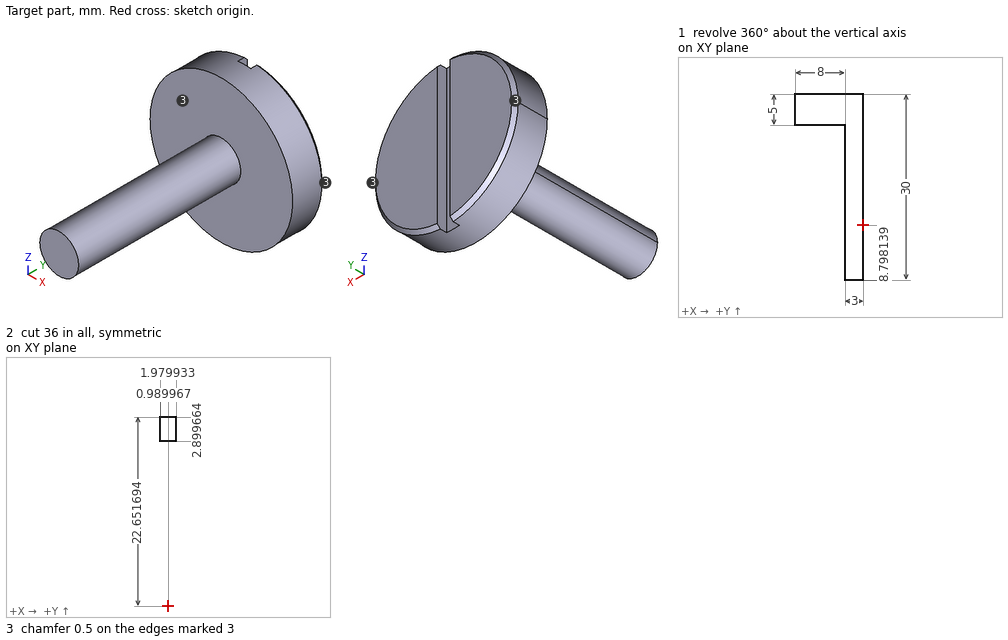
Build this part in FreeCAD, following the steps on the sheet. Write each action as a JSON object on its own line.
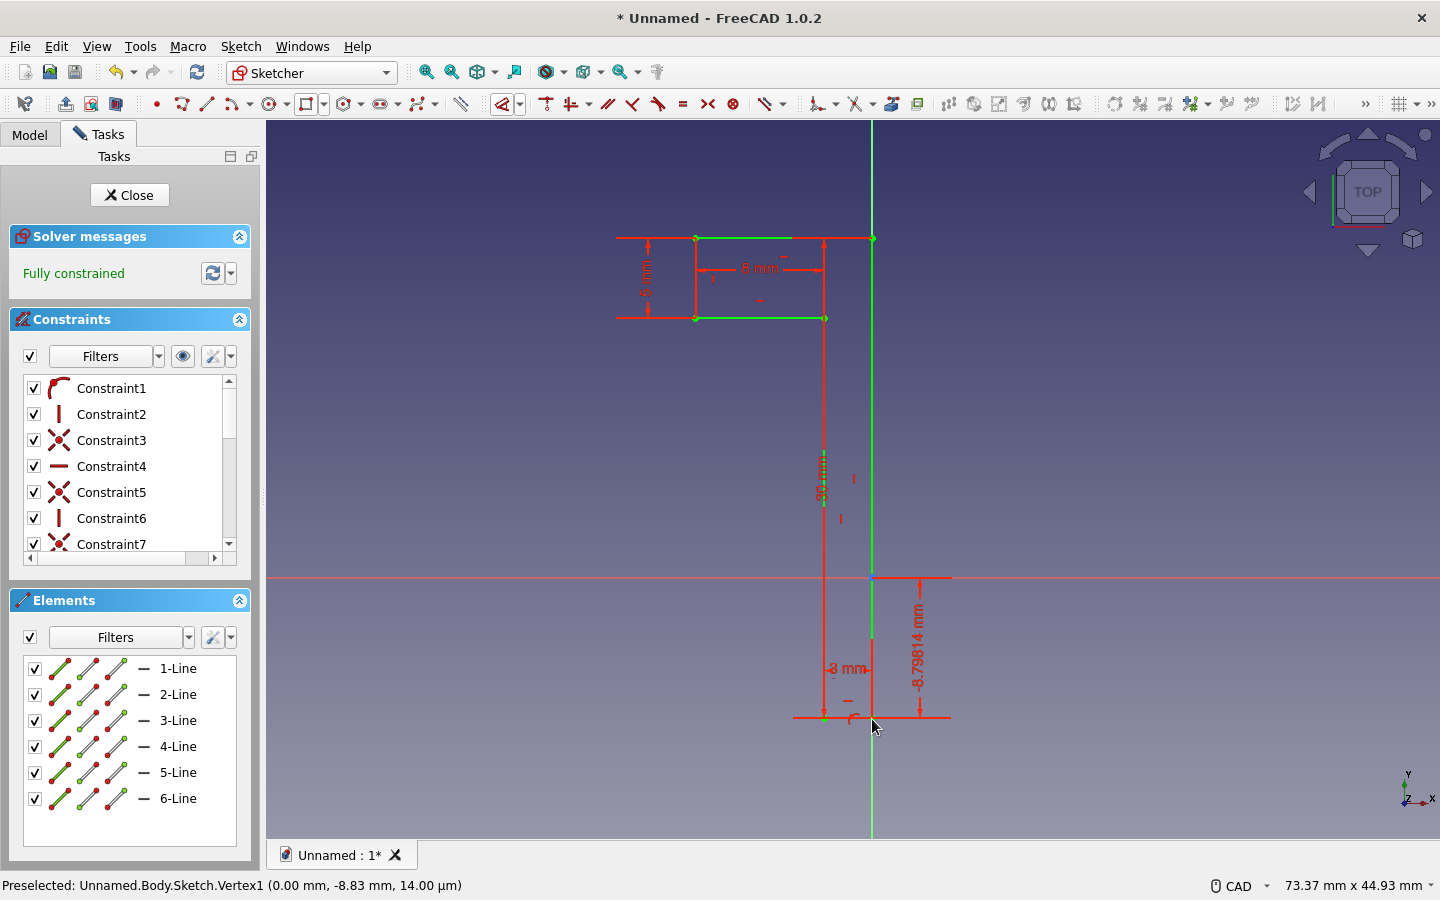
{"action": "left_click", "coordinate": [130, 195]}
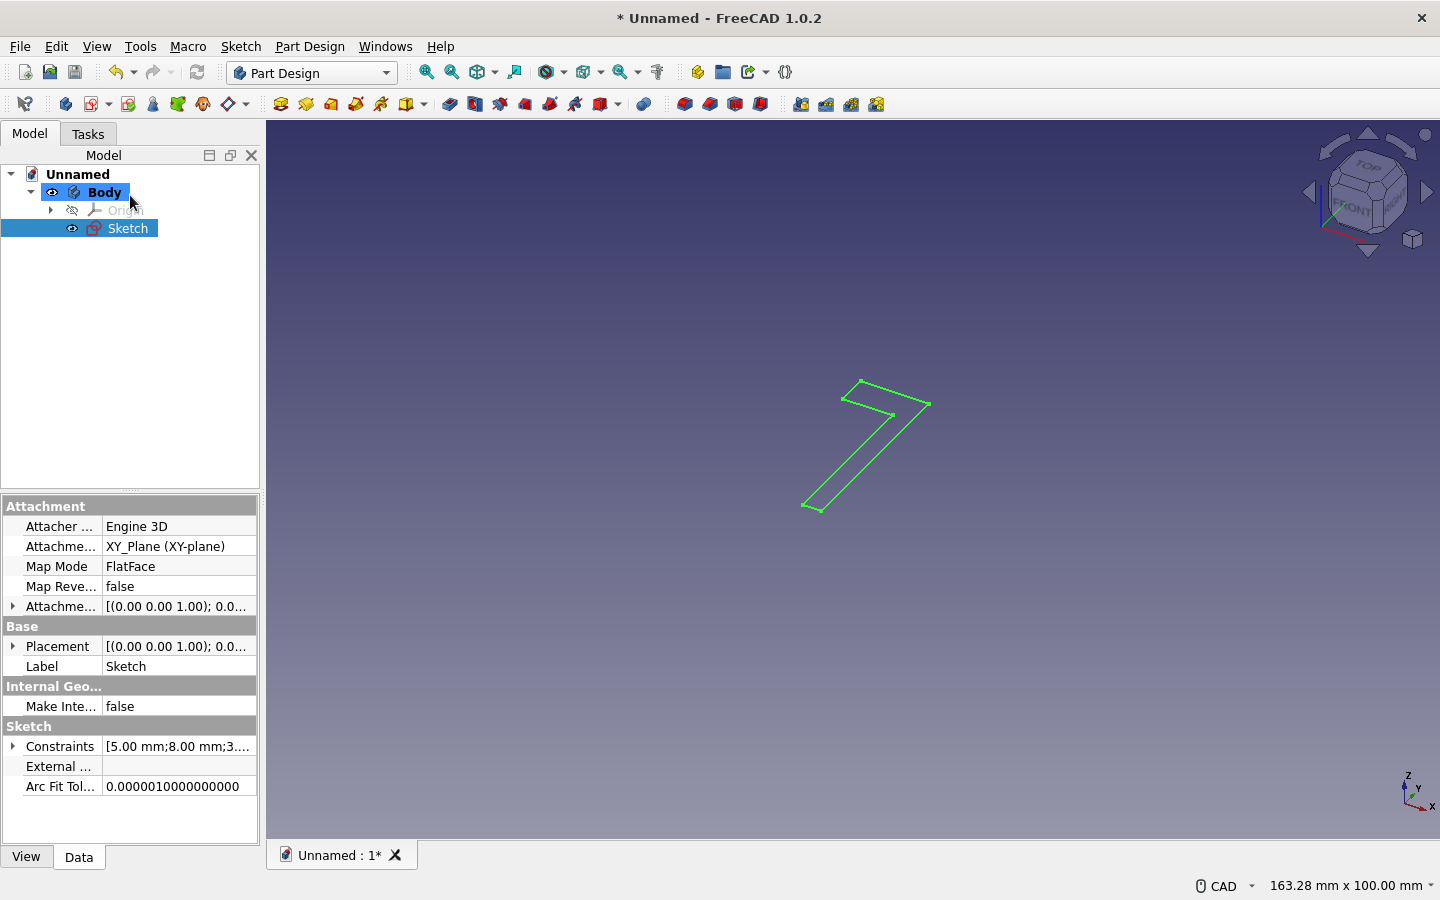
{"action": "left_click", "coordinate": [306, 104]}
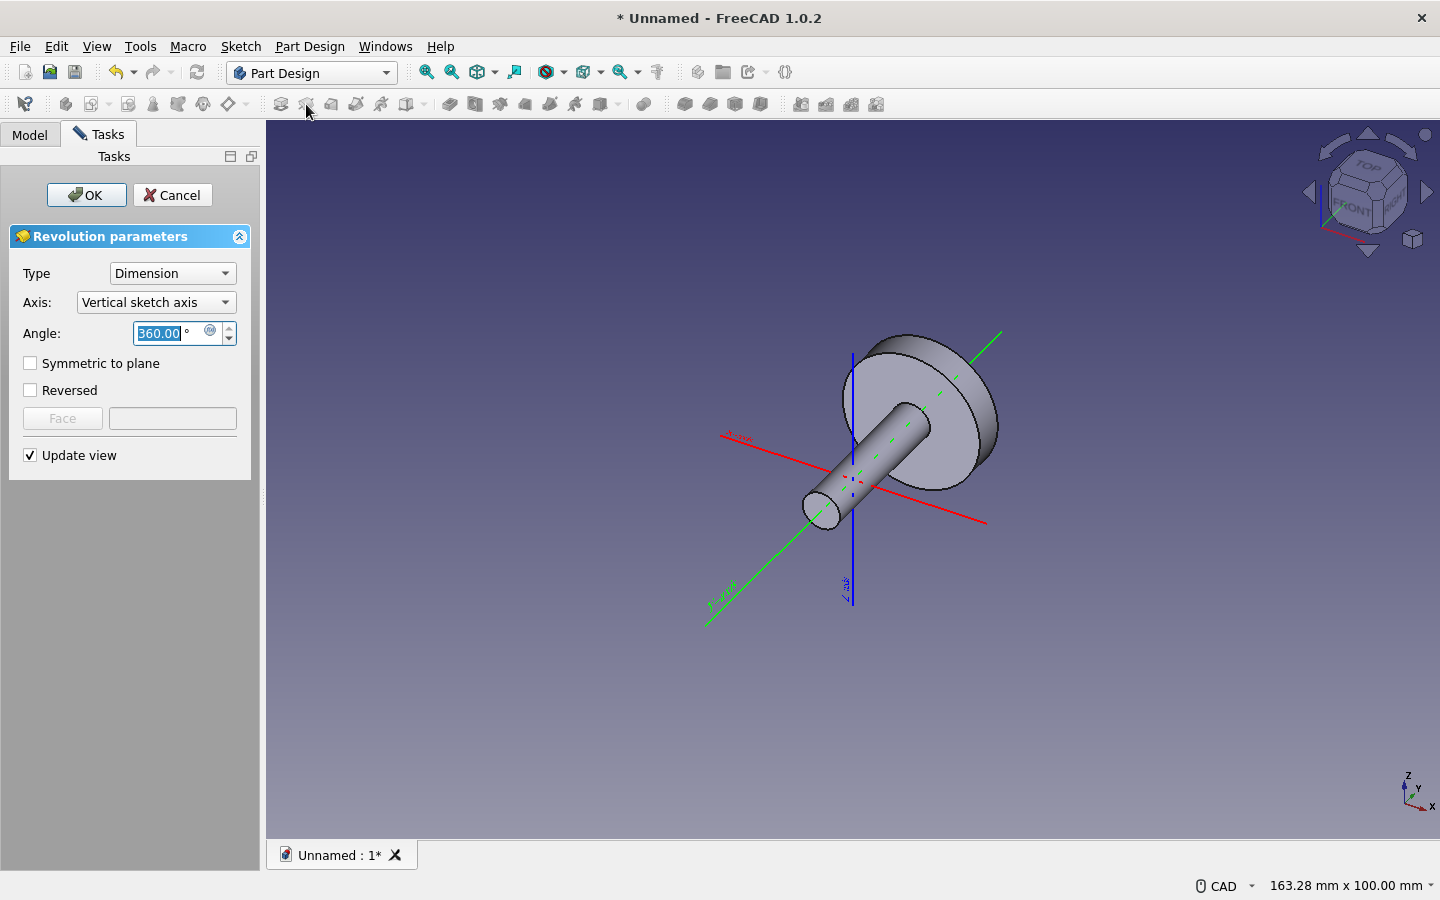
{"action": "left_click", "coordinate": [87, 195]}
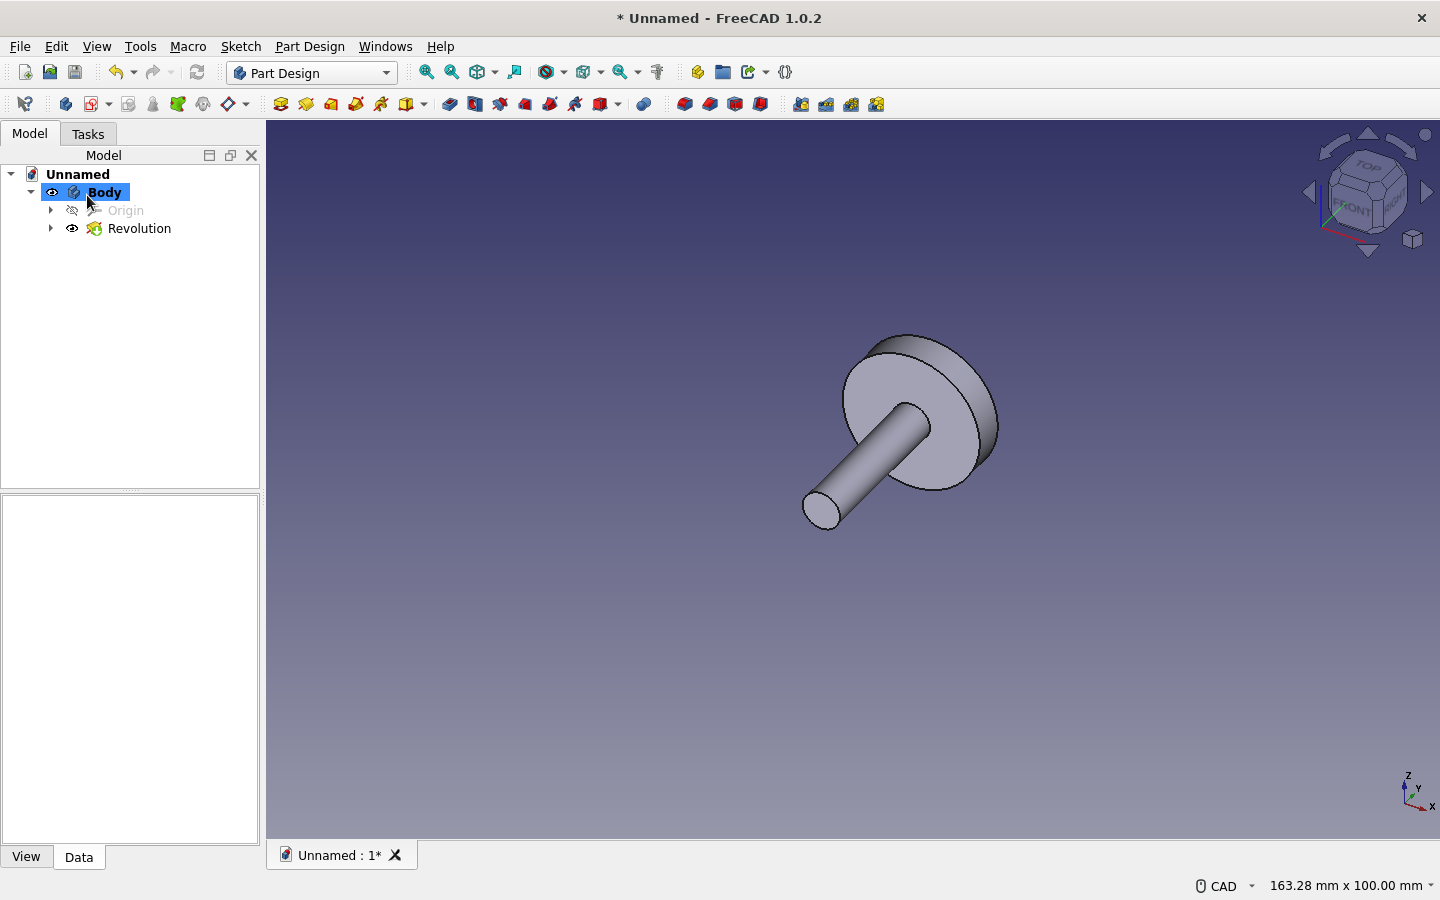
{"action": "left_click", "coordinate": [427, 72]}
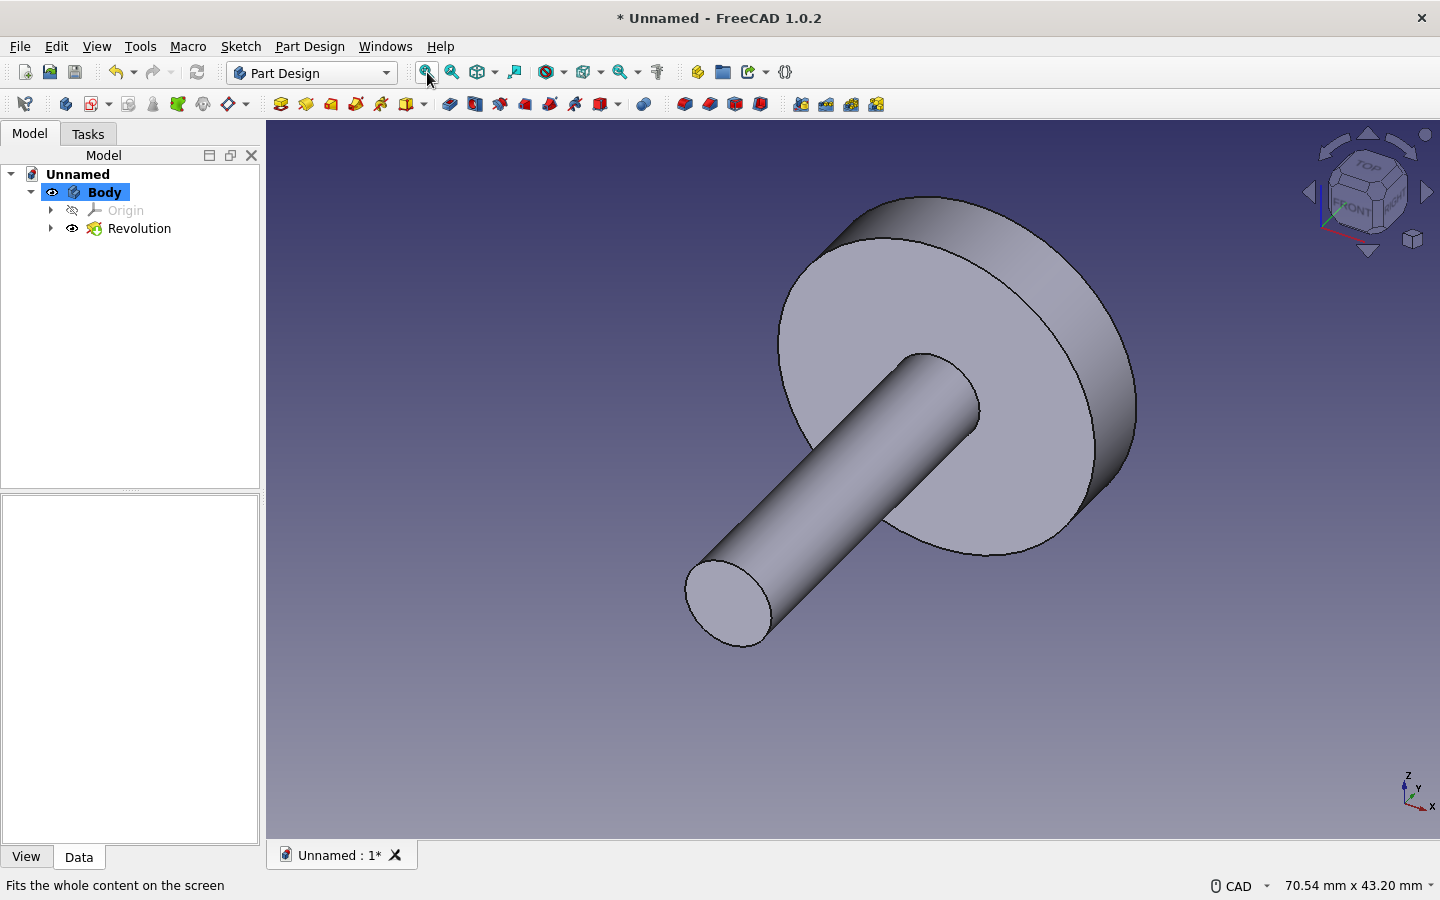
{"action": "left_click", "coordinate": [90, 104]}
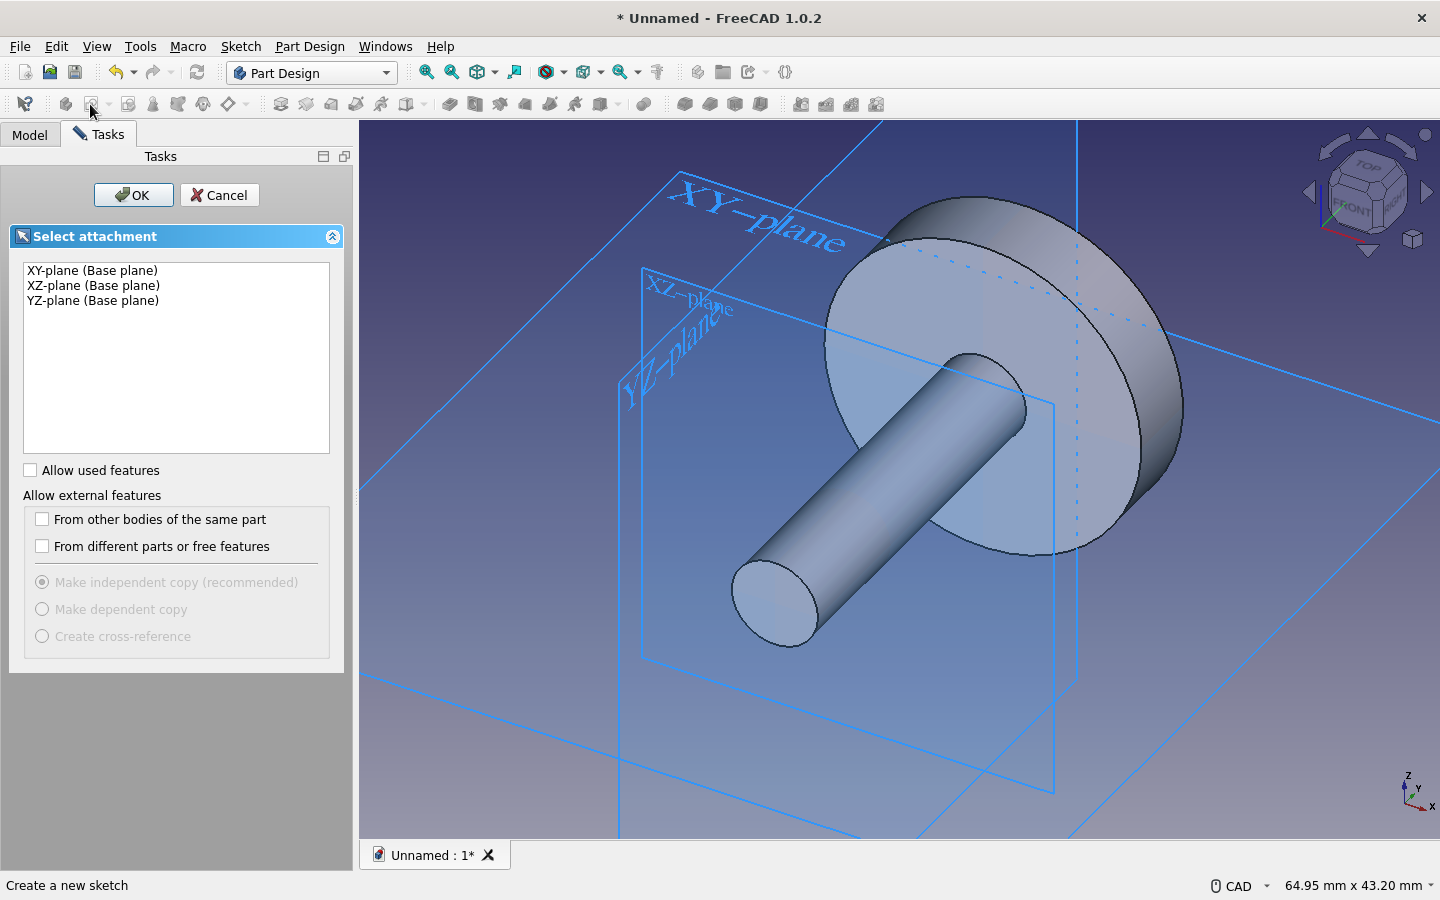
{"action": "left_click", "coordinate": [84, 270]}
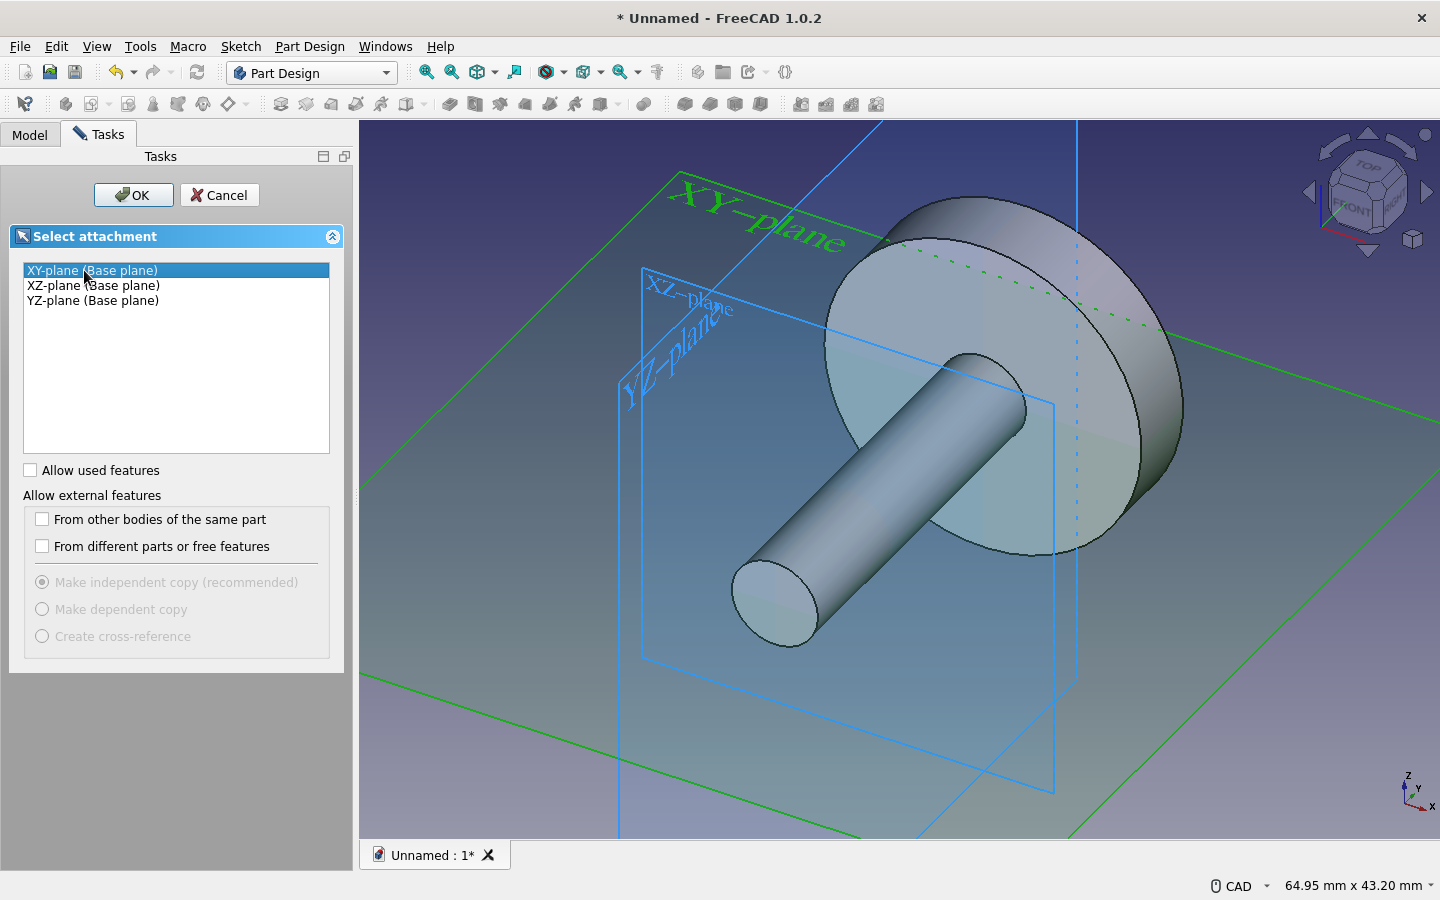
{"action": "left_click", "coordinate": [134, 195]}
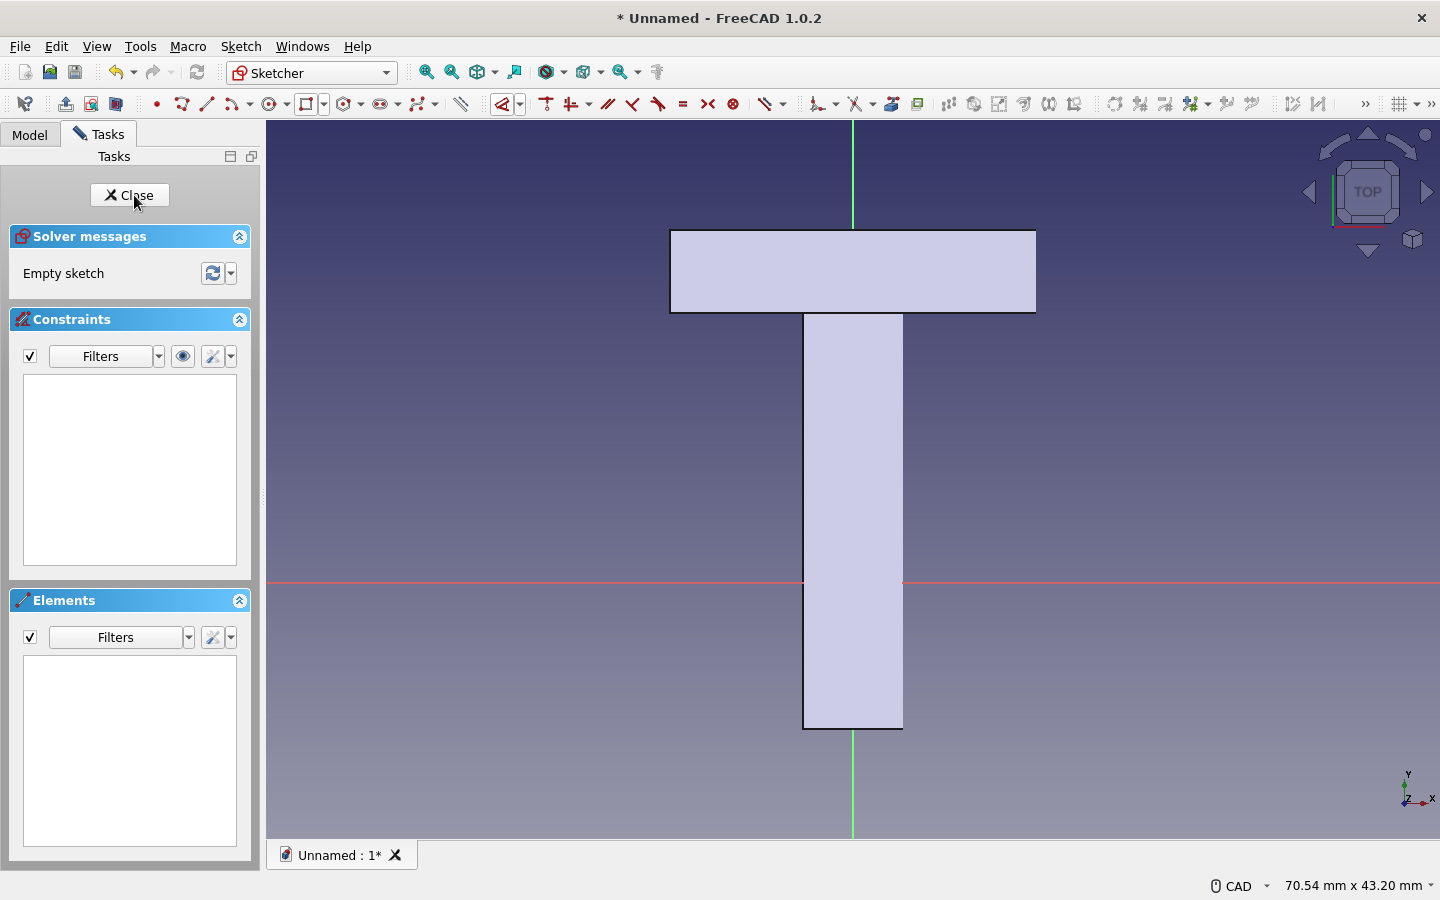
{"action": "left_click", "coordinate": [116, 104]}